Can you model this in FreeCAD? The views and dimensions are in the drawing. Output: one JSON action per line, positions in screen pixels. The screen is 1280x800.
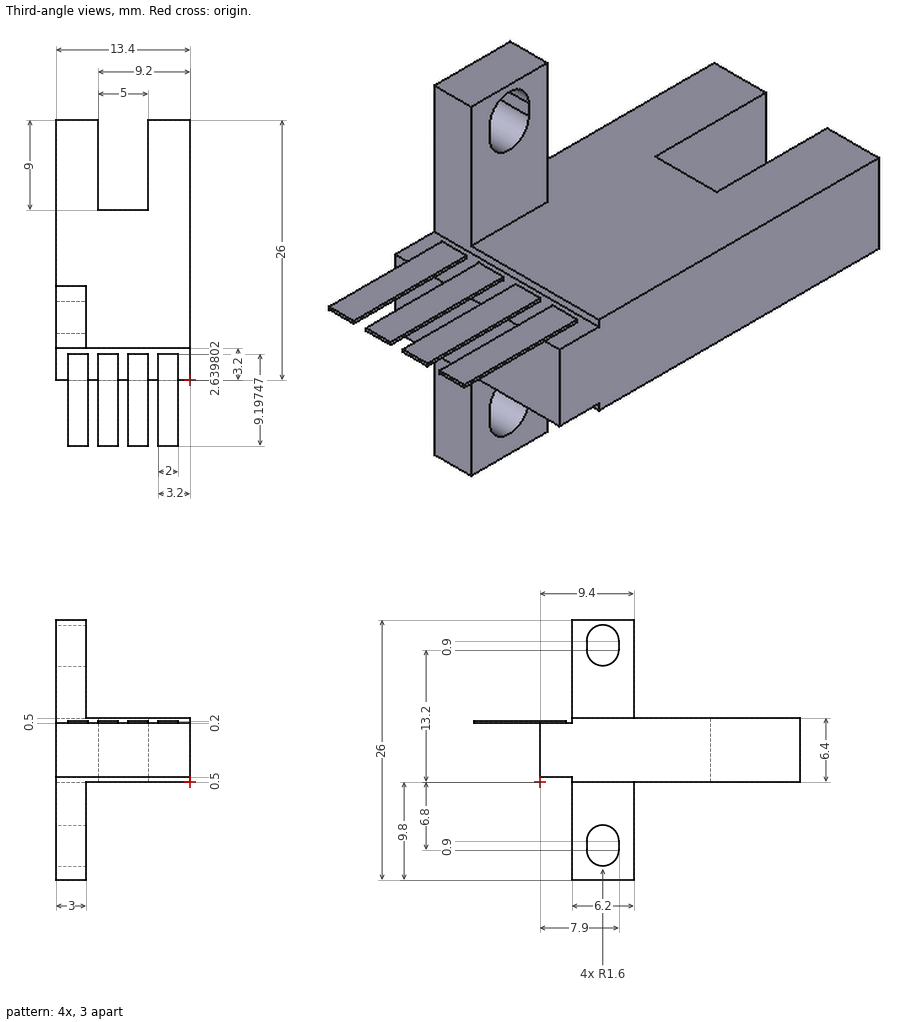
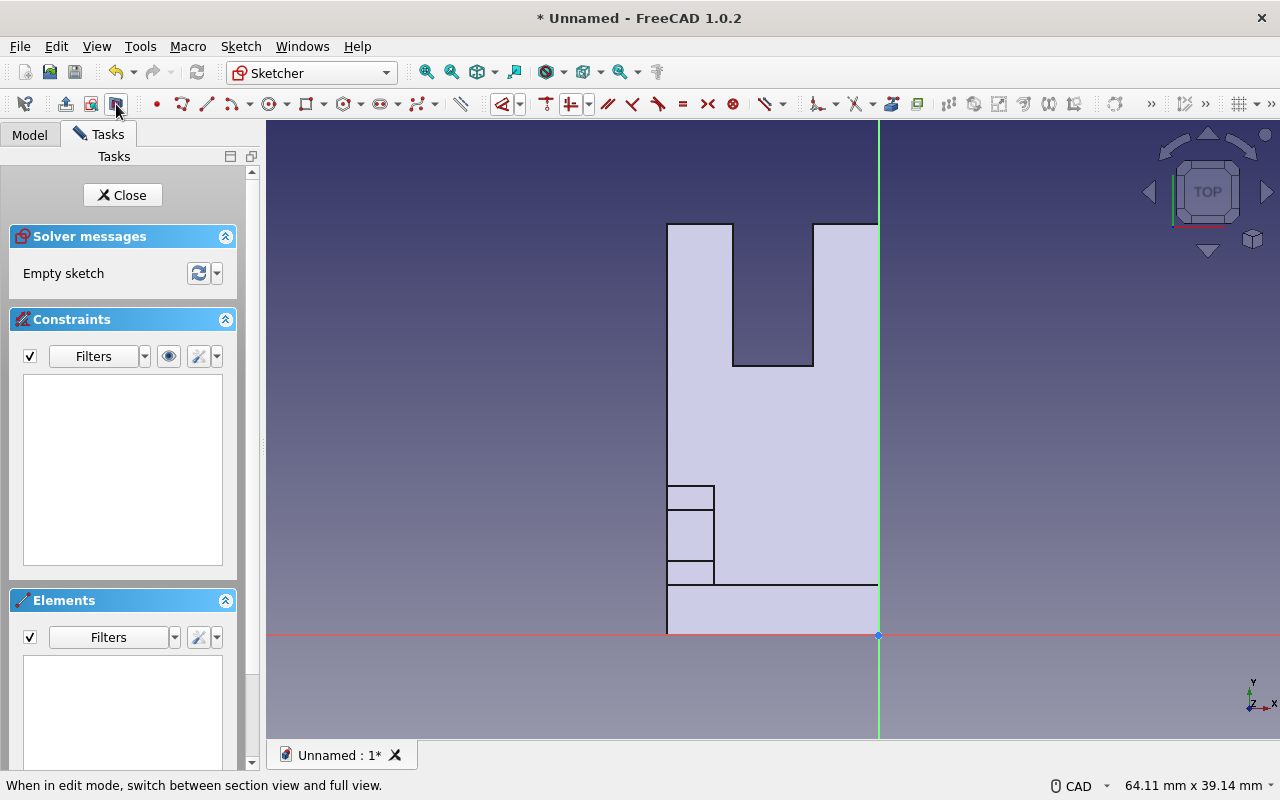
{"action": "scroll", "coordinate": [704, 430], "scroll_direction": "down", "scroll_amount": 5}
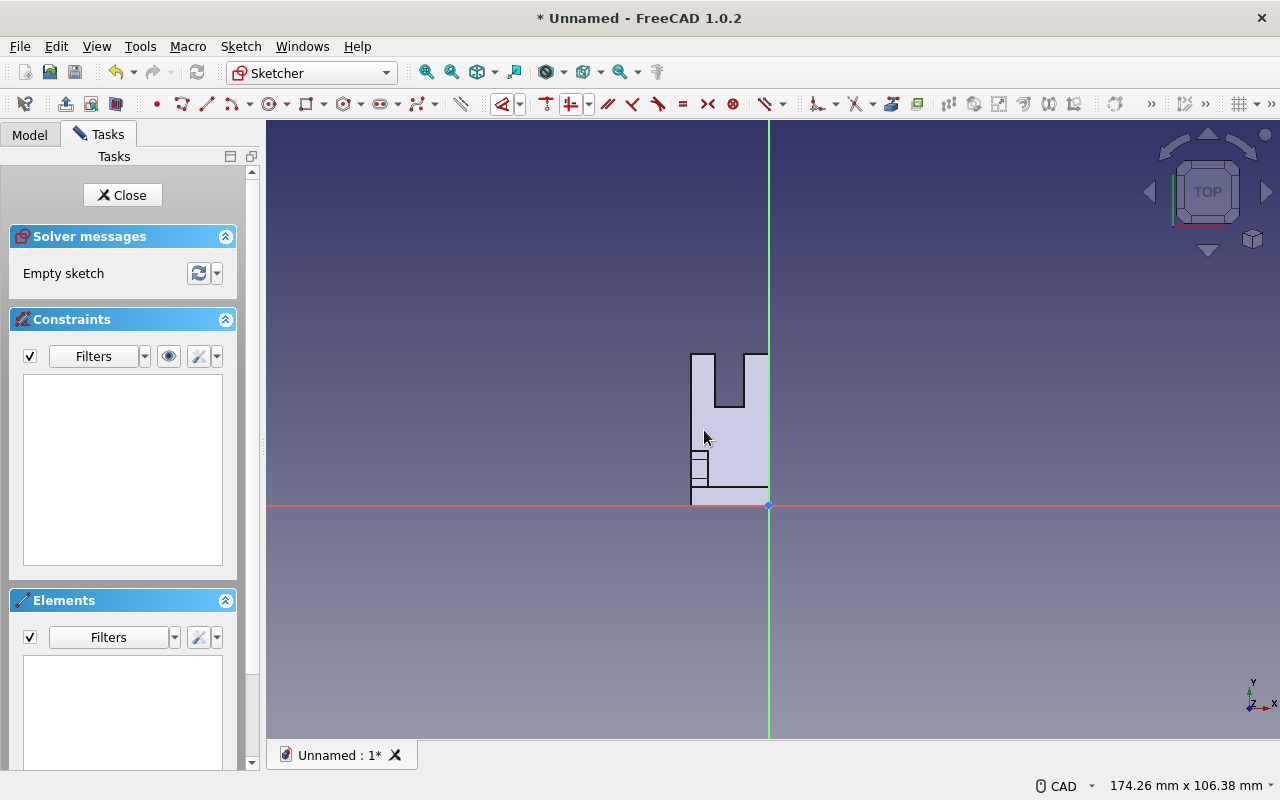
{"action": "scroll", "coordinate": [768, 531], "scroll_direction": "up", "scroll_amount": 10}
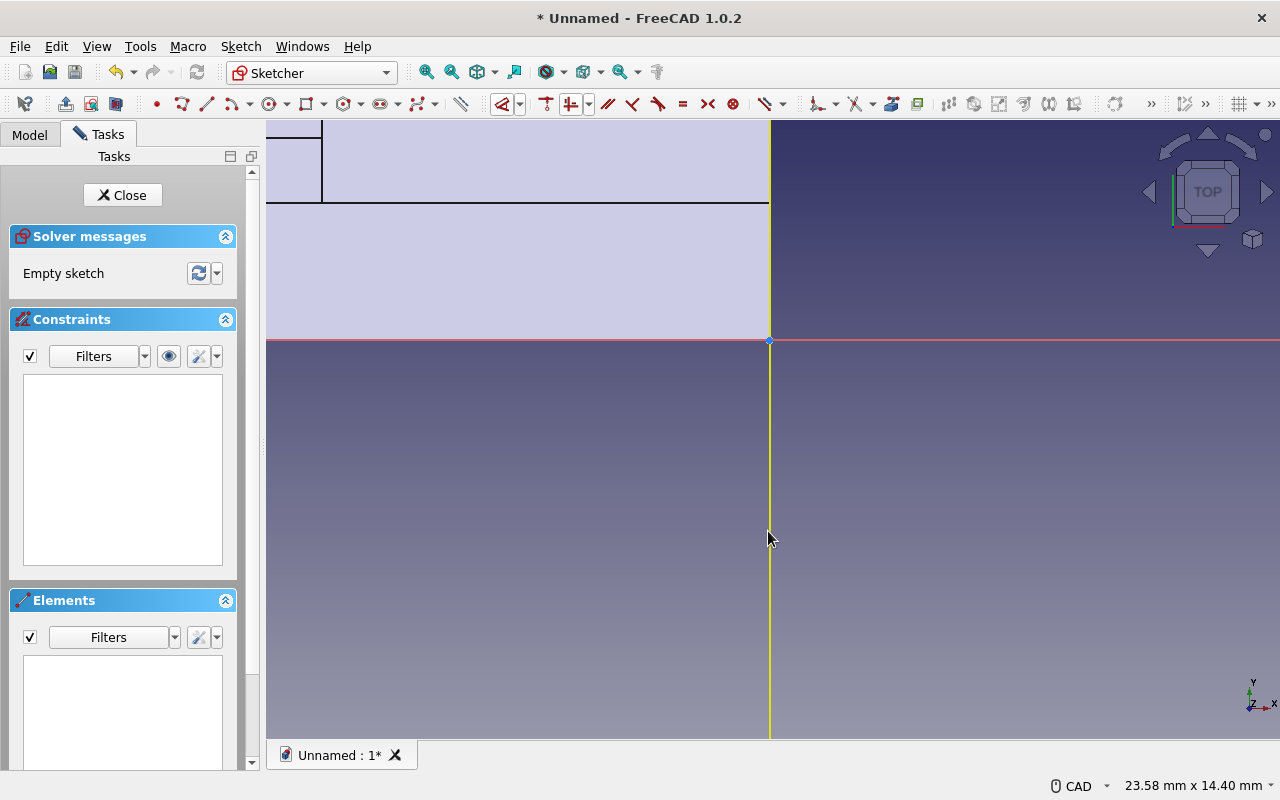
{"action": "left_click", "coordinate": [306, 104]}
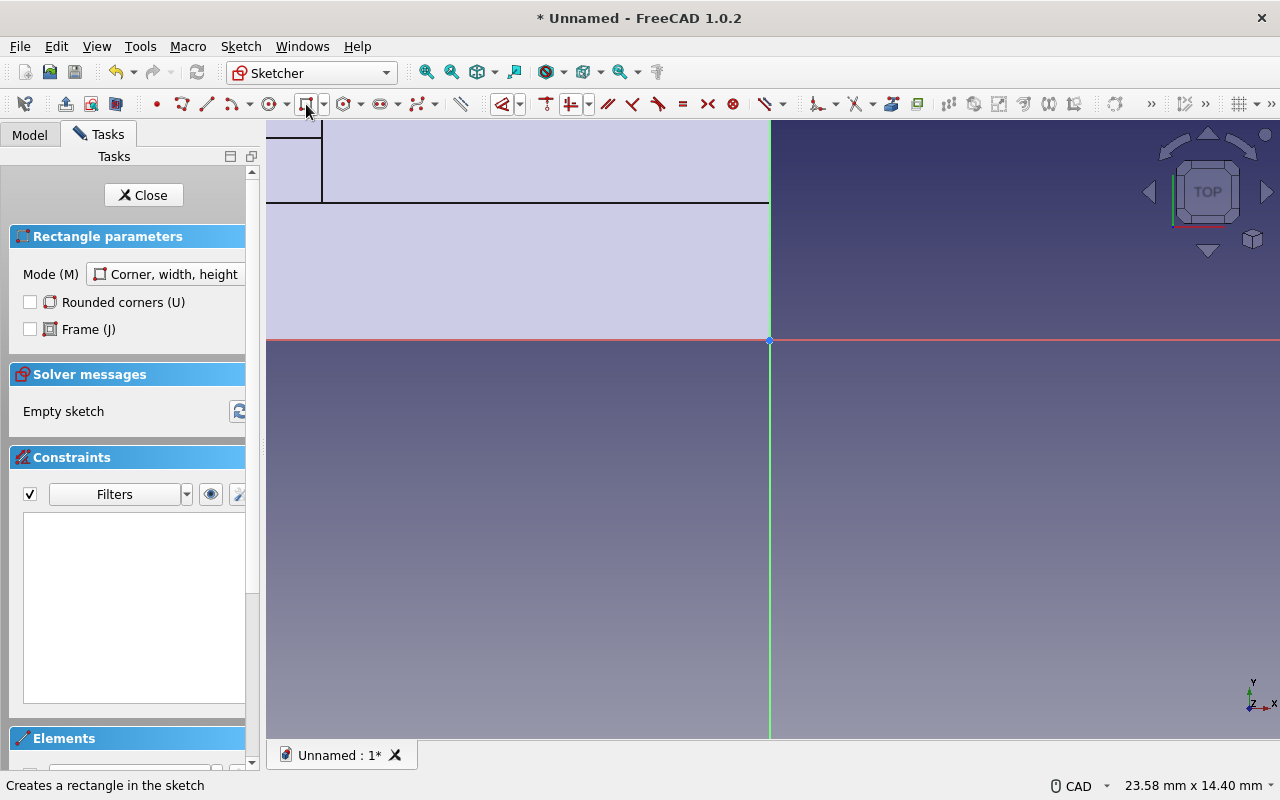
{"action": "left_click", "coordinate": [632, 227]}
{"action": "left_click", "coordinate": [718, 622]}
{"action": "key", "text": "Escape"}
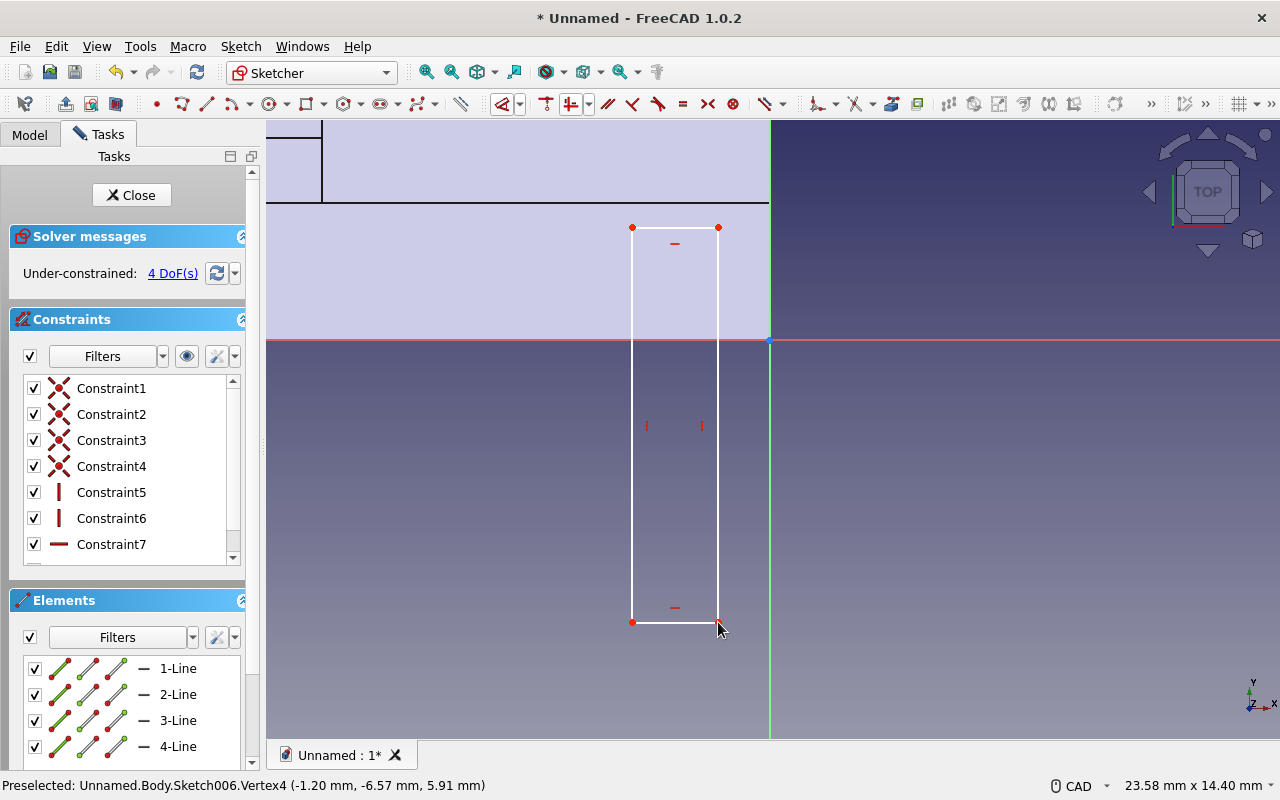
{"action": "left_click", "coordinate": [658, 623]}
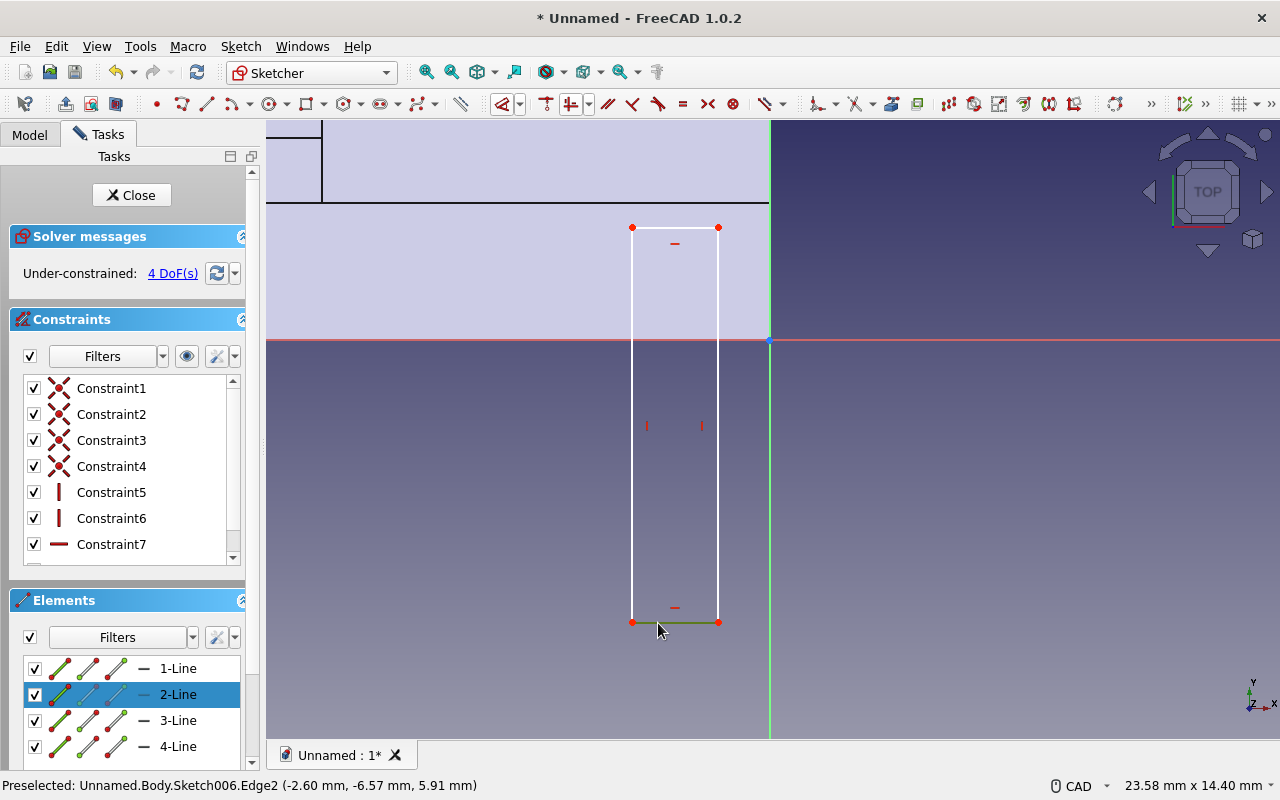
{"action": "left_click", "coordinate": [520, 104]}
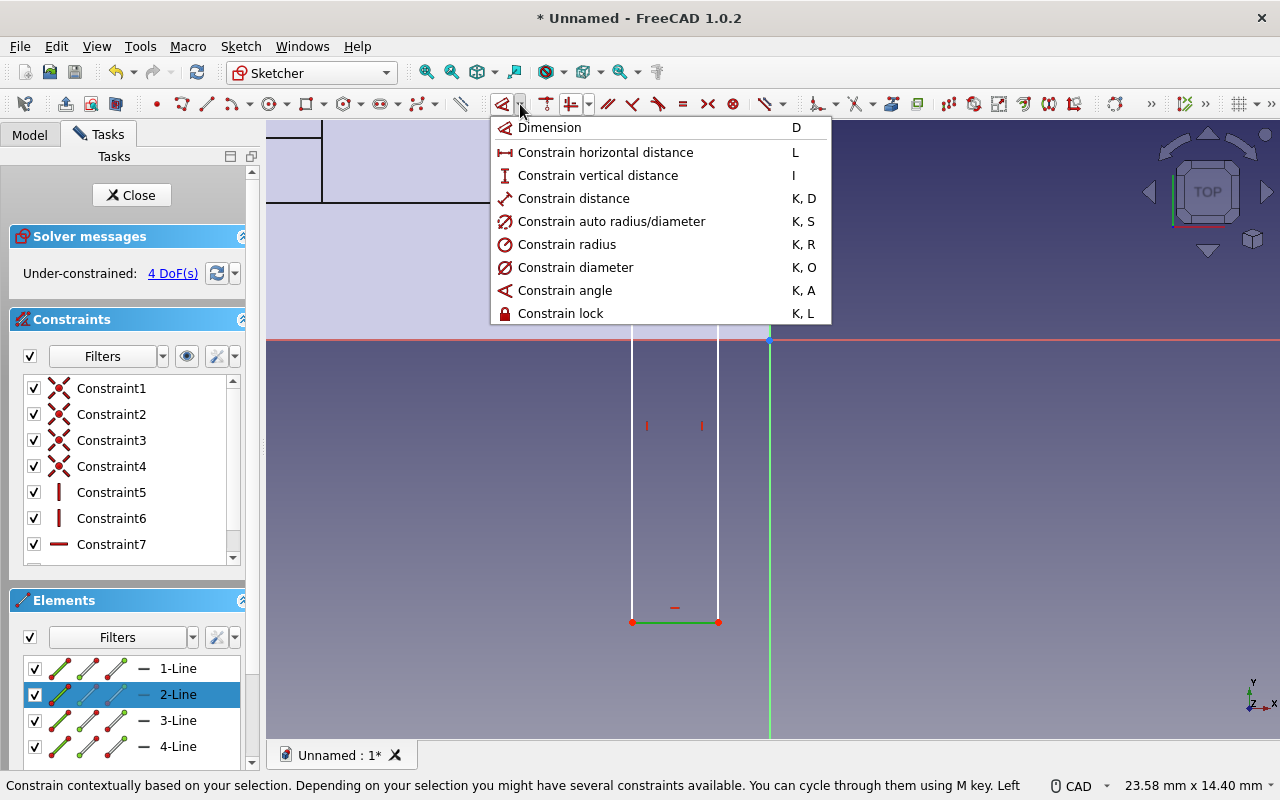
{"action": "left_click", "coordinate": [661, 152]}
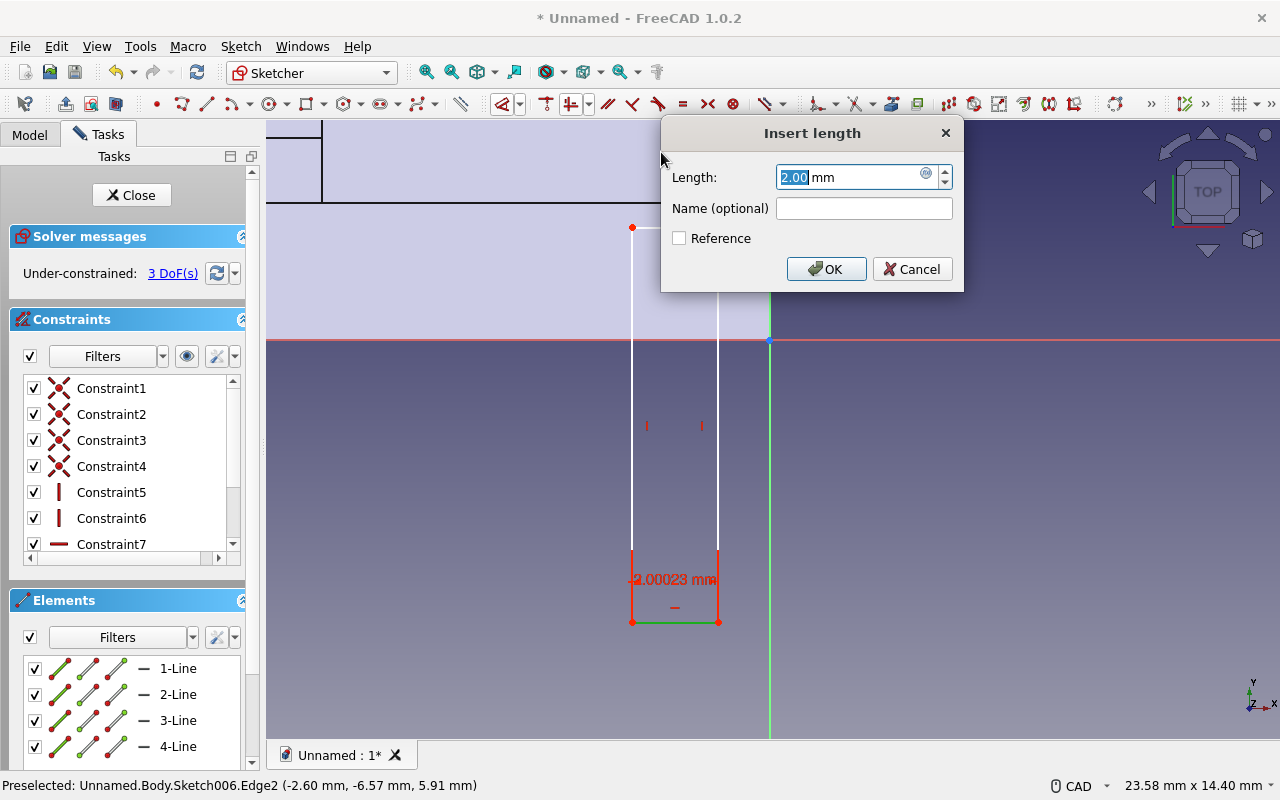
{"action": "type", "text": "2"}
{"action": "key", "text": "Return"}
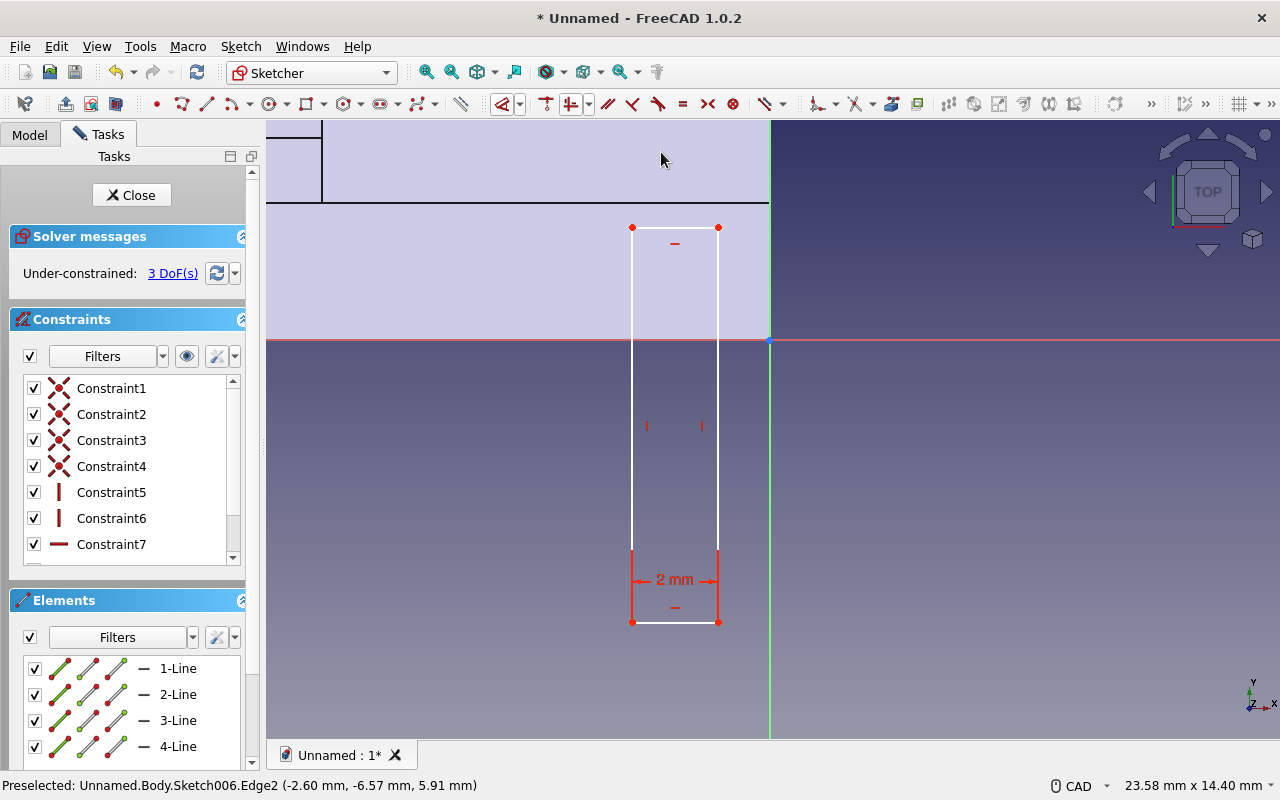
{"action": "left_click", "coordinate": [632, 228]}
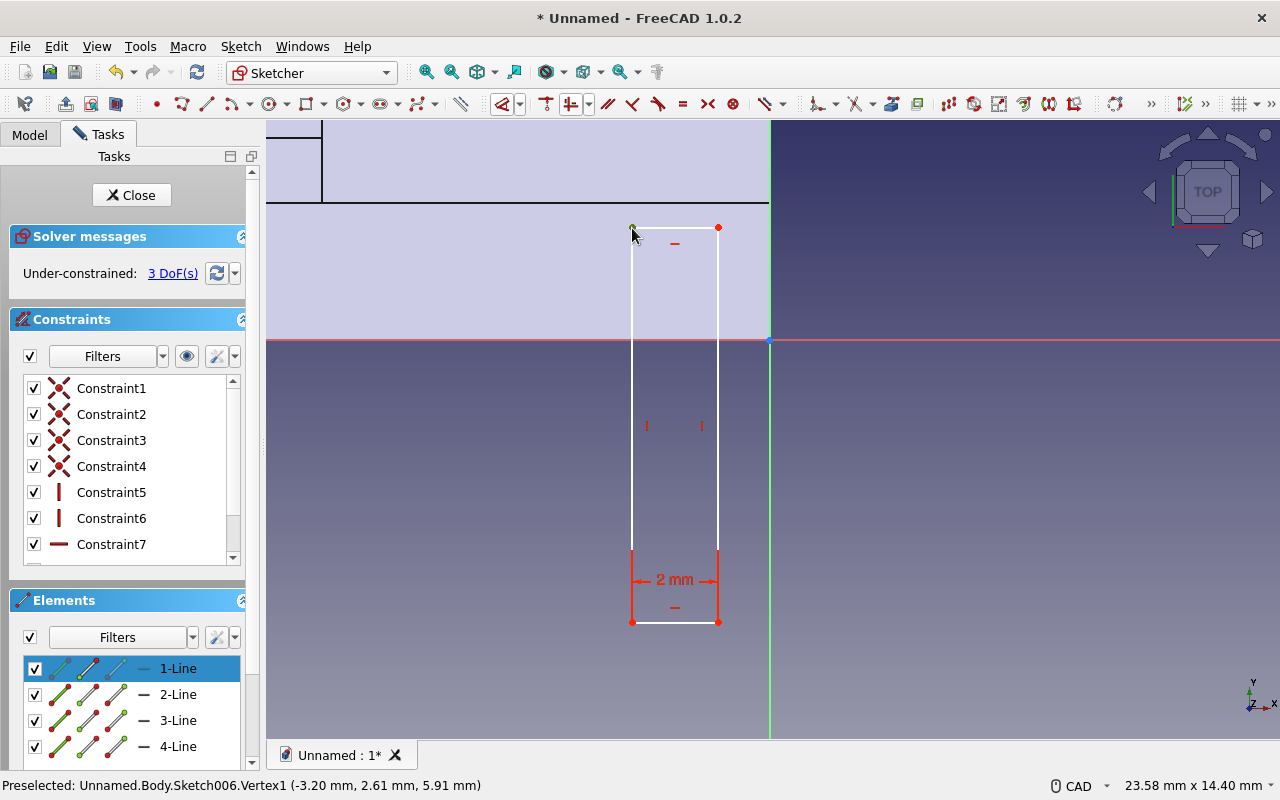
{"action": "left_click", "coordinate": [520, 104]}